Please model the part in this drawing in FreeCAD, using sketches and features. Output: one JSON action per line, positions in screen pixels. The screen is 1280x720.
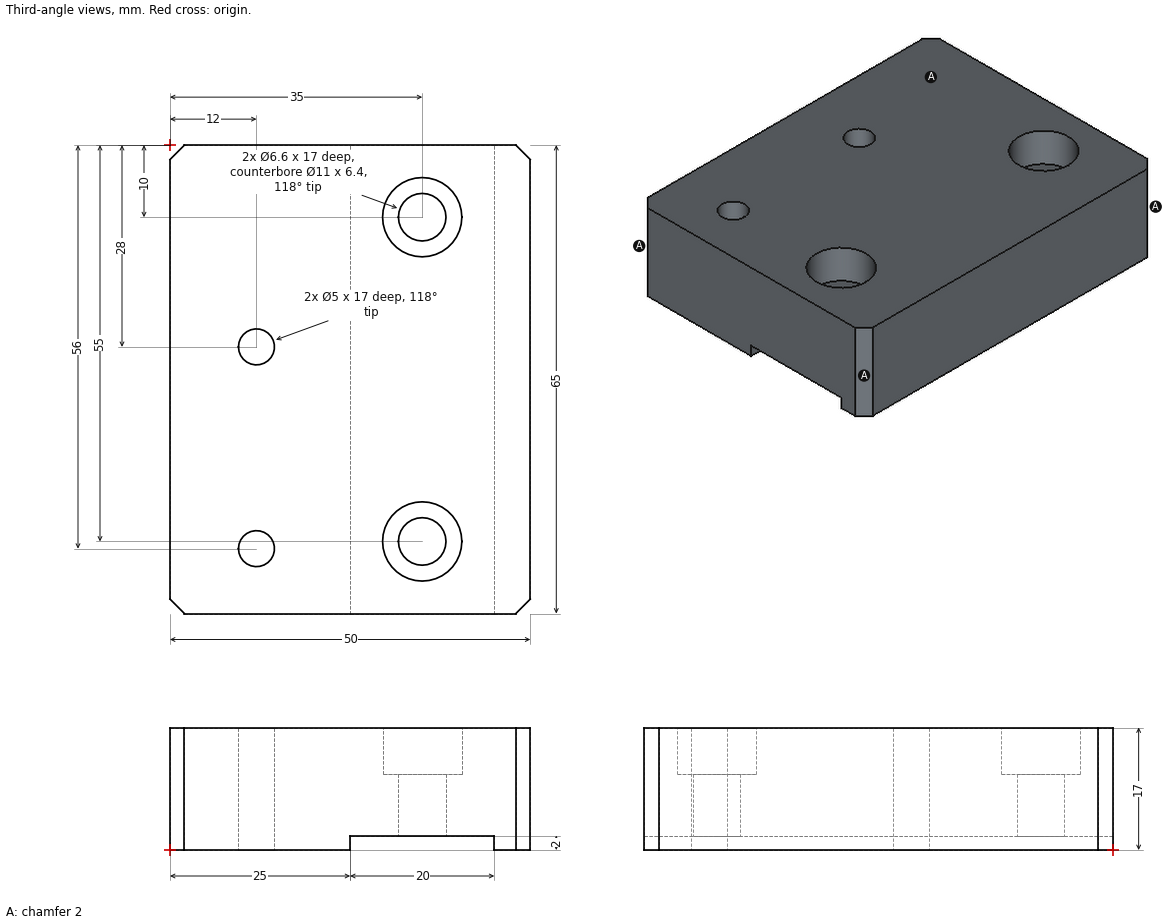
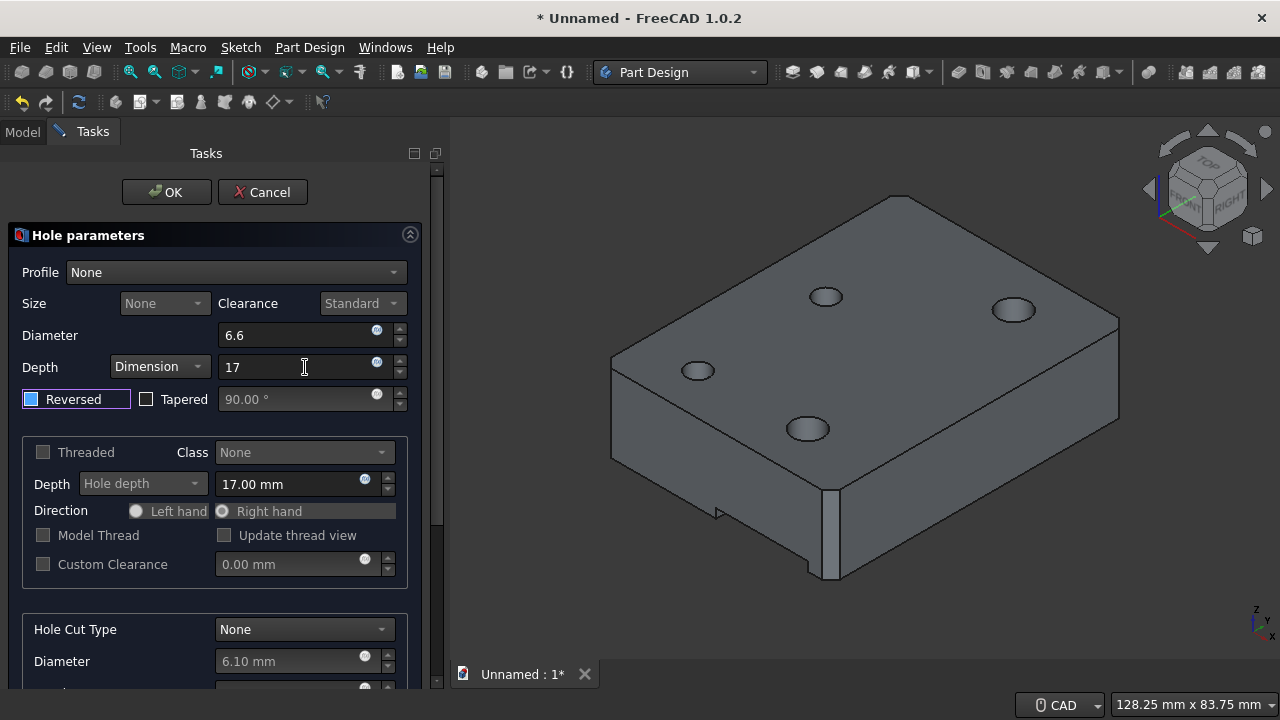
{"action": "left_click", "coordinate": [306, 630]}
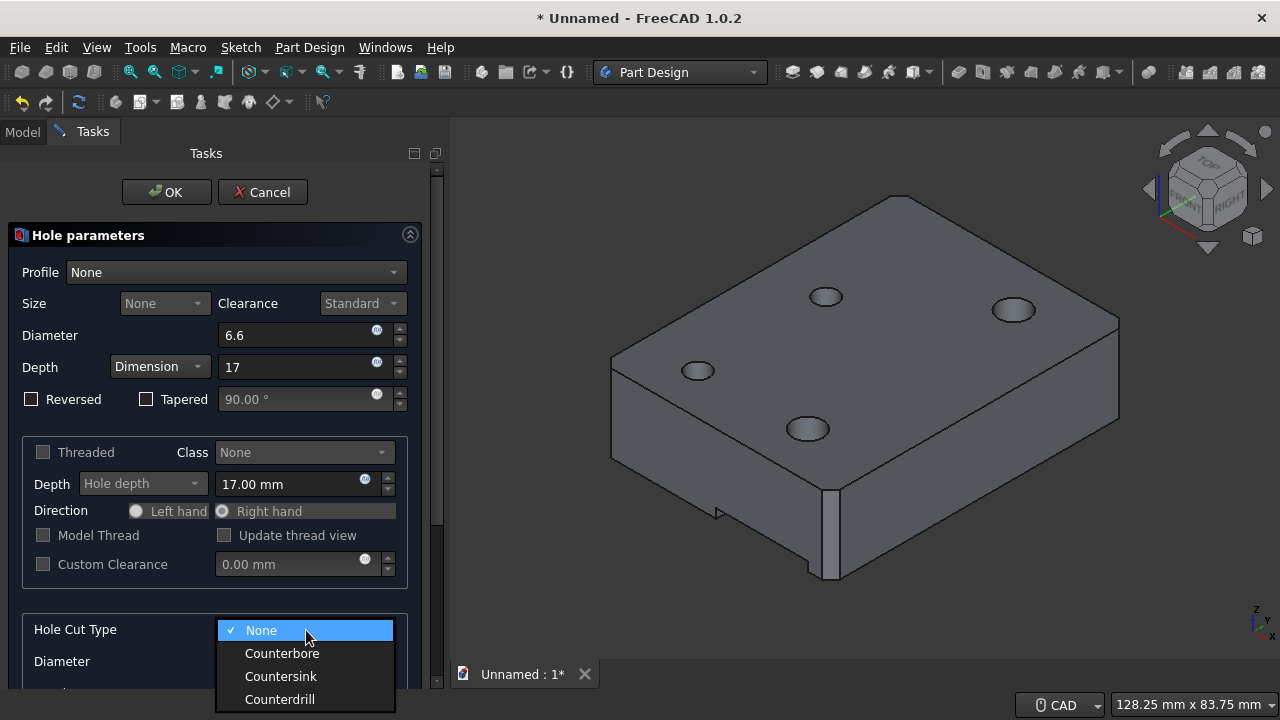
{"action": "left_click", "coordinate": [304, 654]}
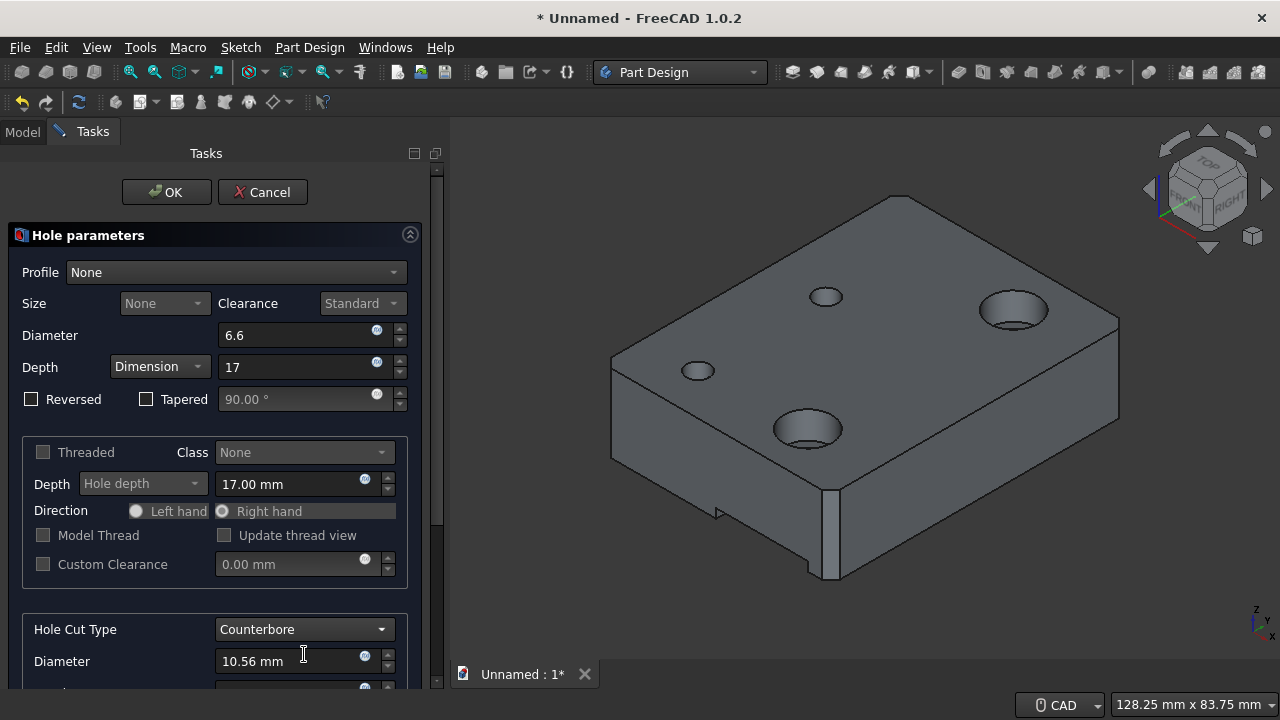
{"action": "triple_click", "coordinate": [298, 661]}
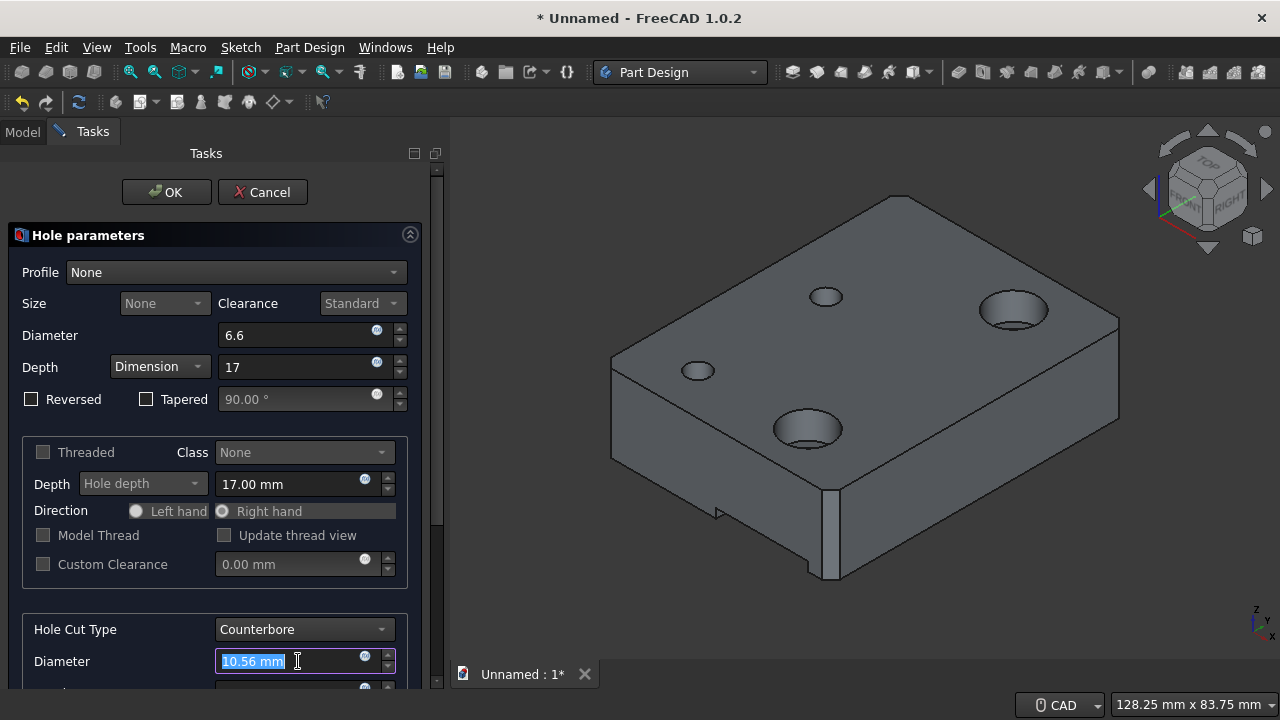
{"action": "type", "text": "11"}
{"action": "key", "text": "Tab"}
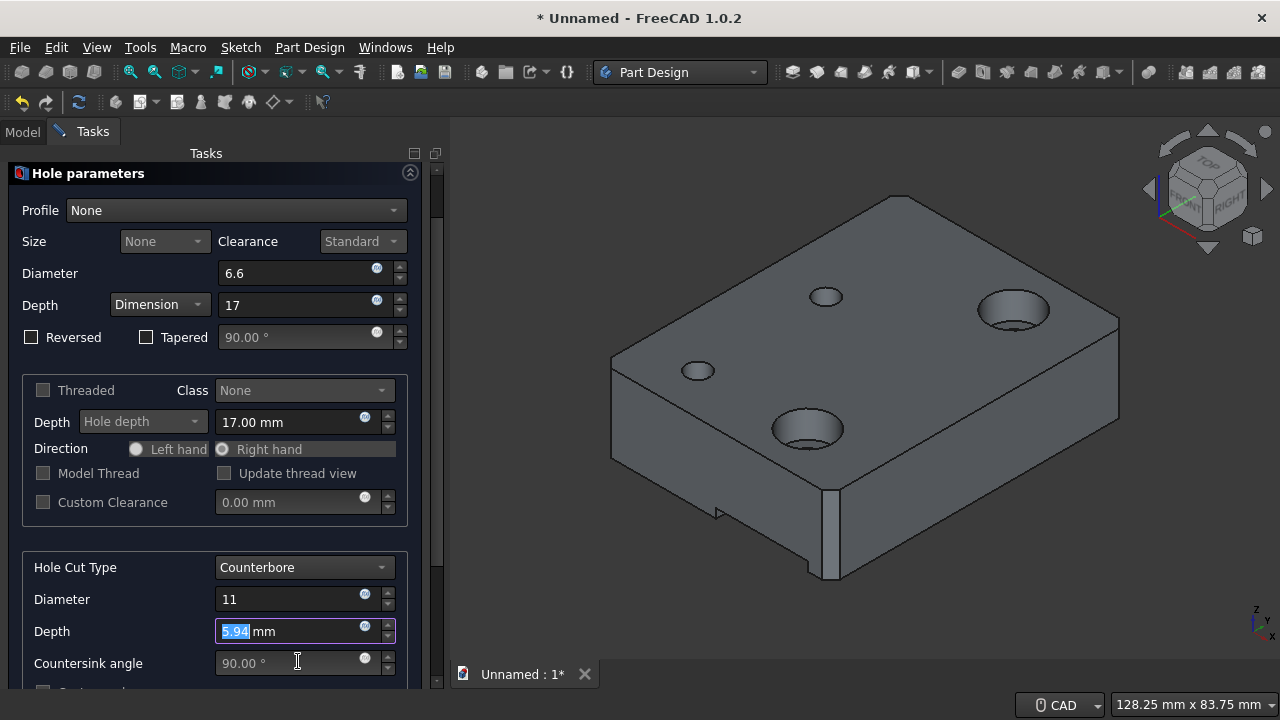
{"action": "type", "text": "6.4"}
{"action": "key", "text": "Tab"}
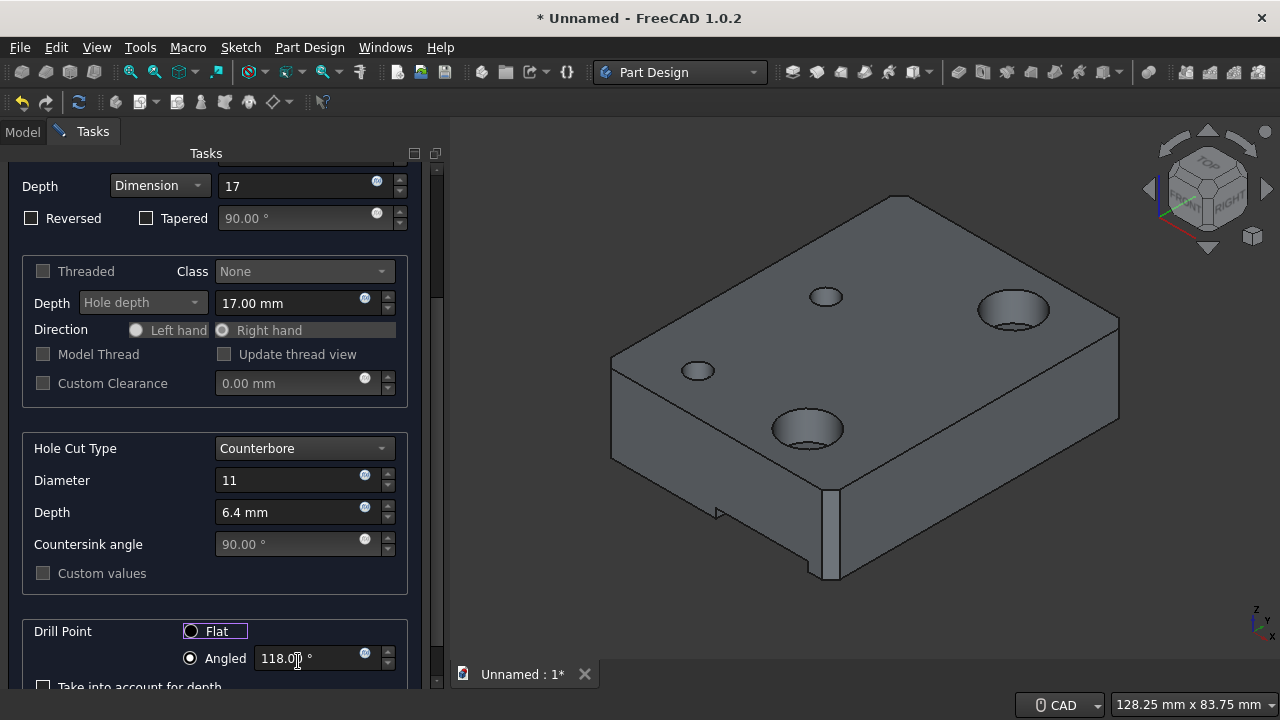
{"action": "scroll", "coordinate": [437, 426], "scroll_direction": "up", "scroll_amount": 4}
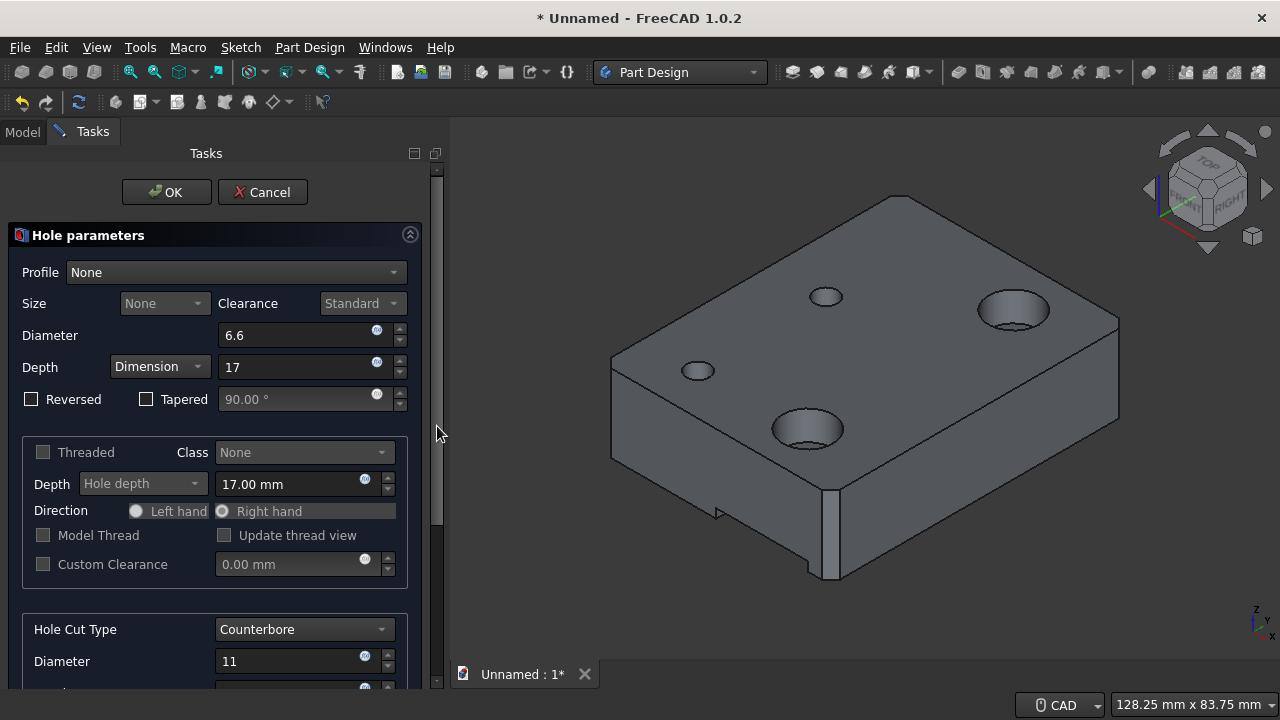
{"action": "left_click", "coordinate": [167, 192]}